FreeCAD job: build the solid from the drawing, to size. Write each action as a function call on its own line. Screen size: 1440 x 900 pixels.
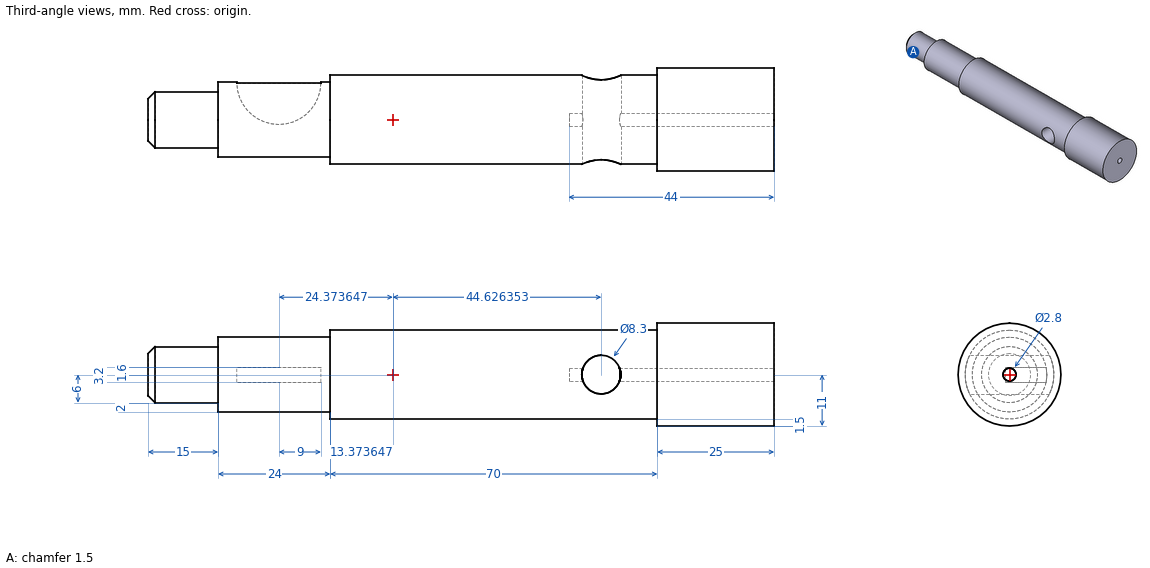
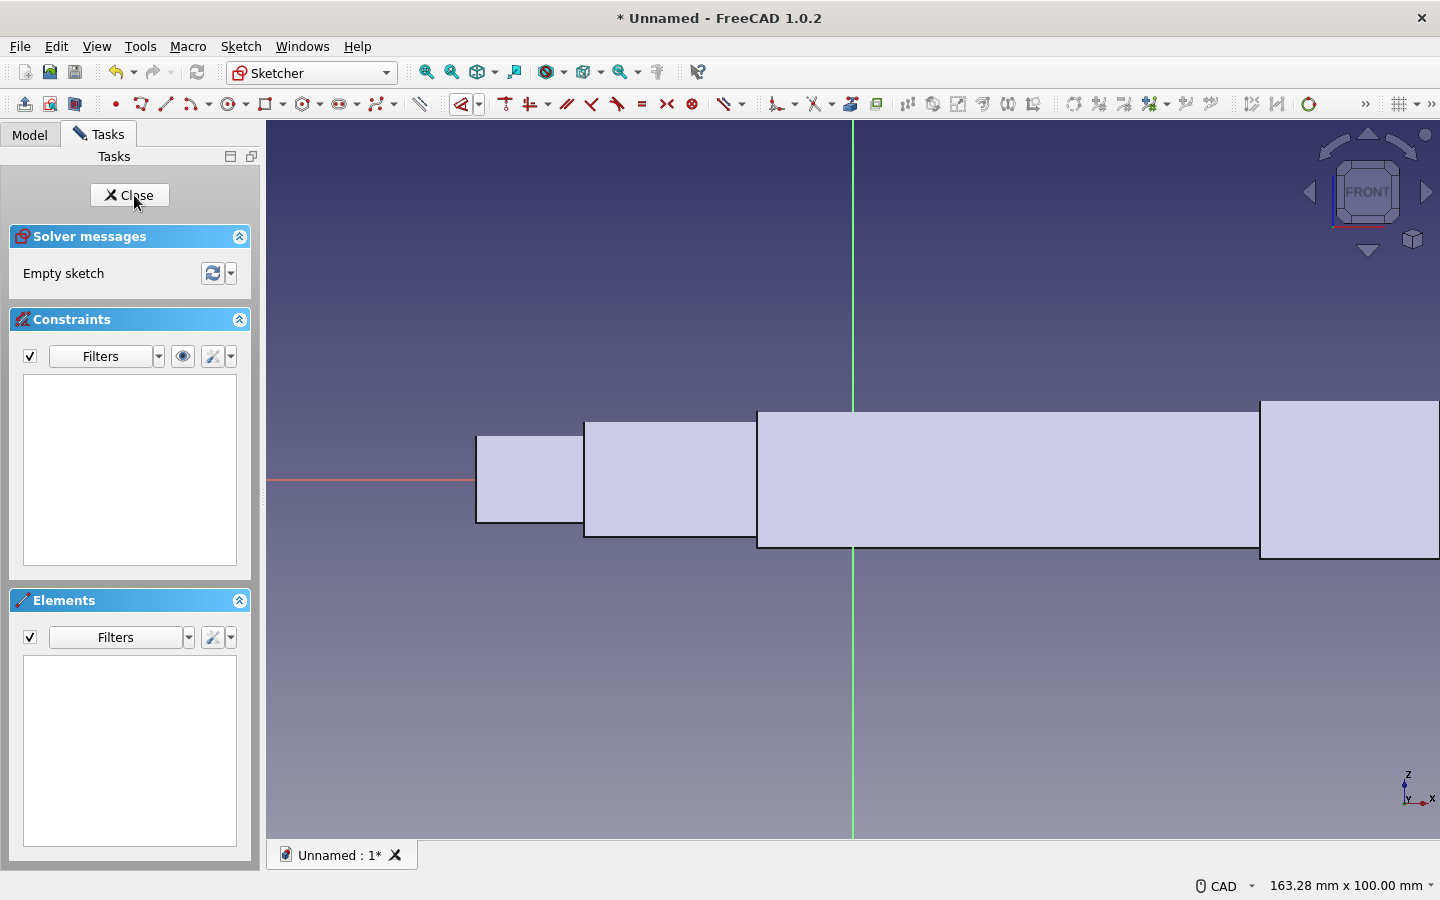
click(75, 104)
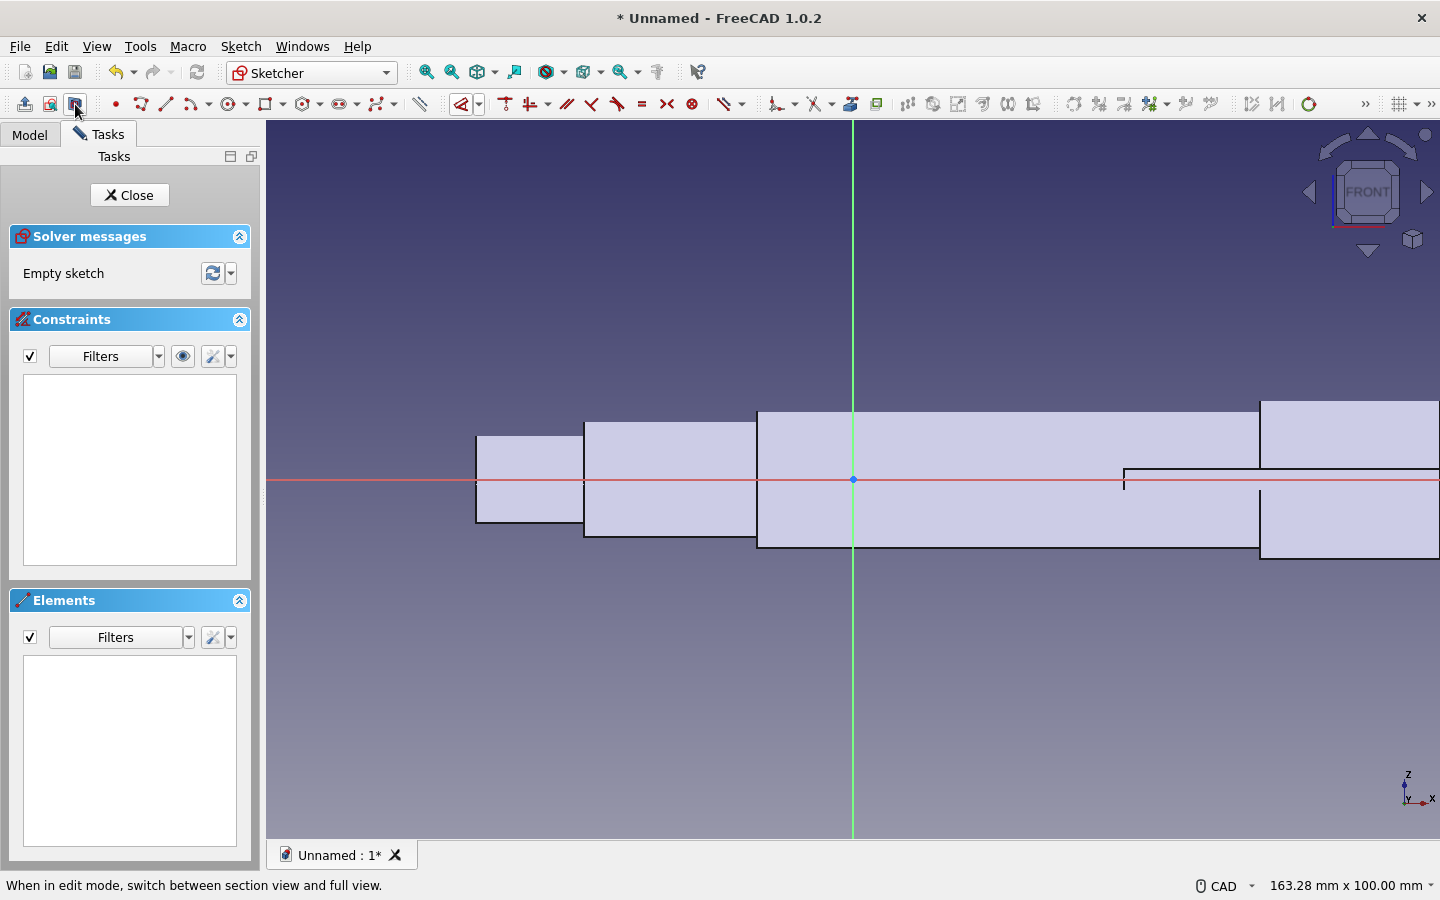
scroll(1235, 480, up, 10)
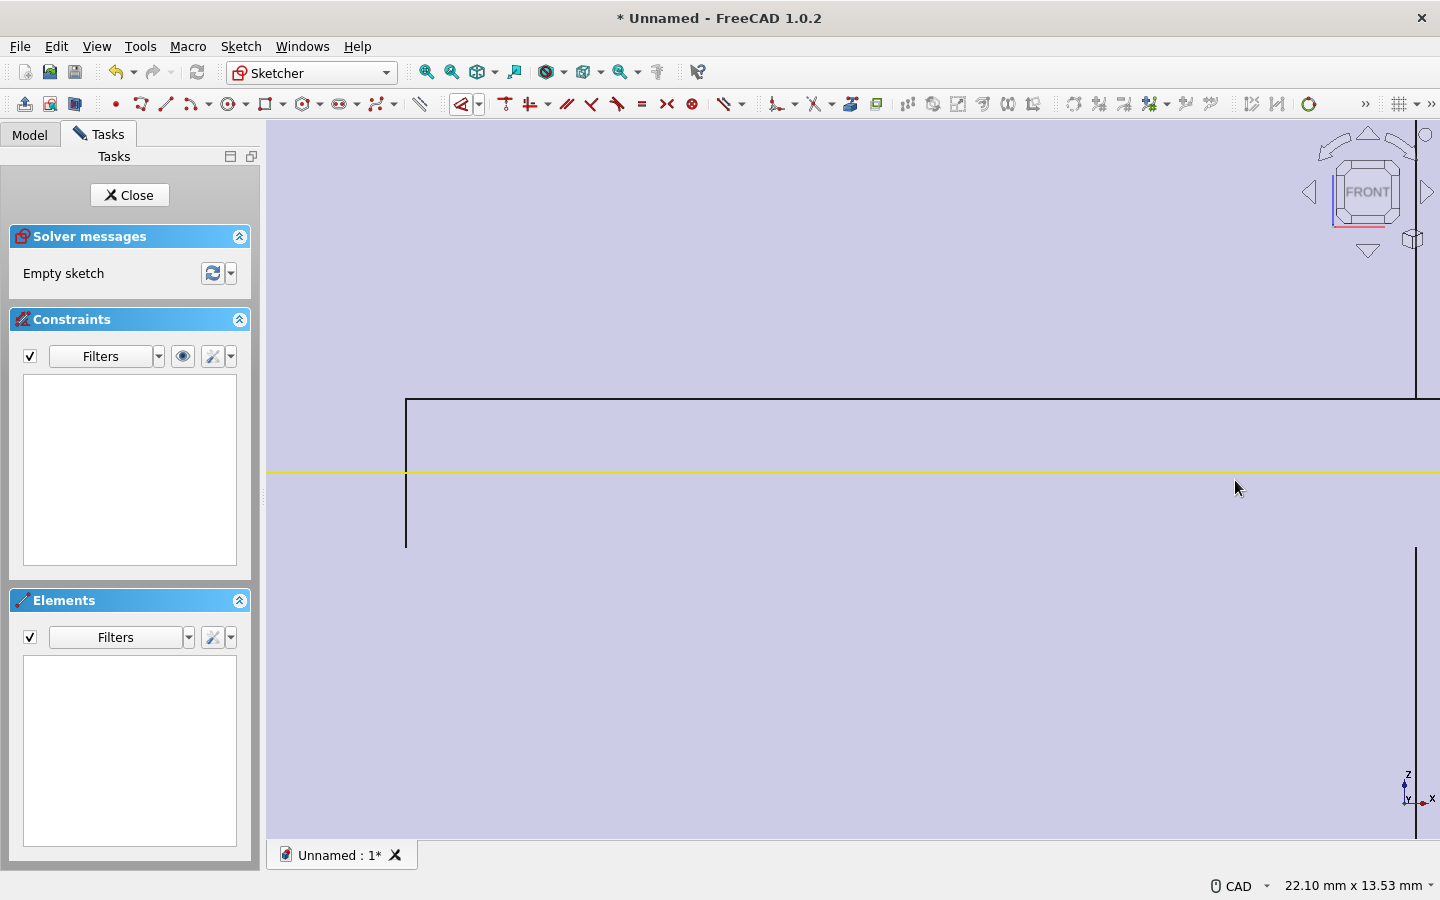
click(228, 104)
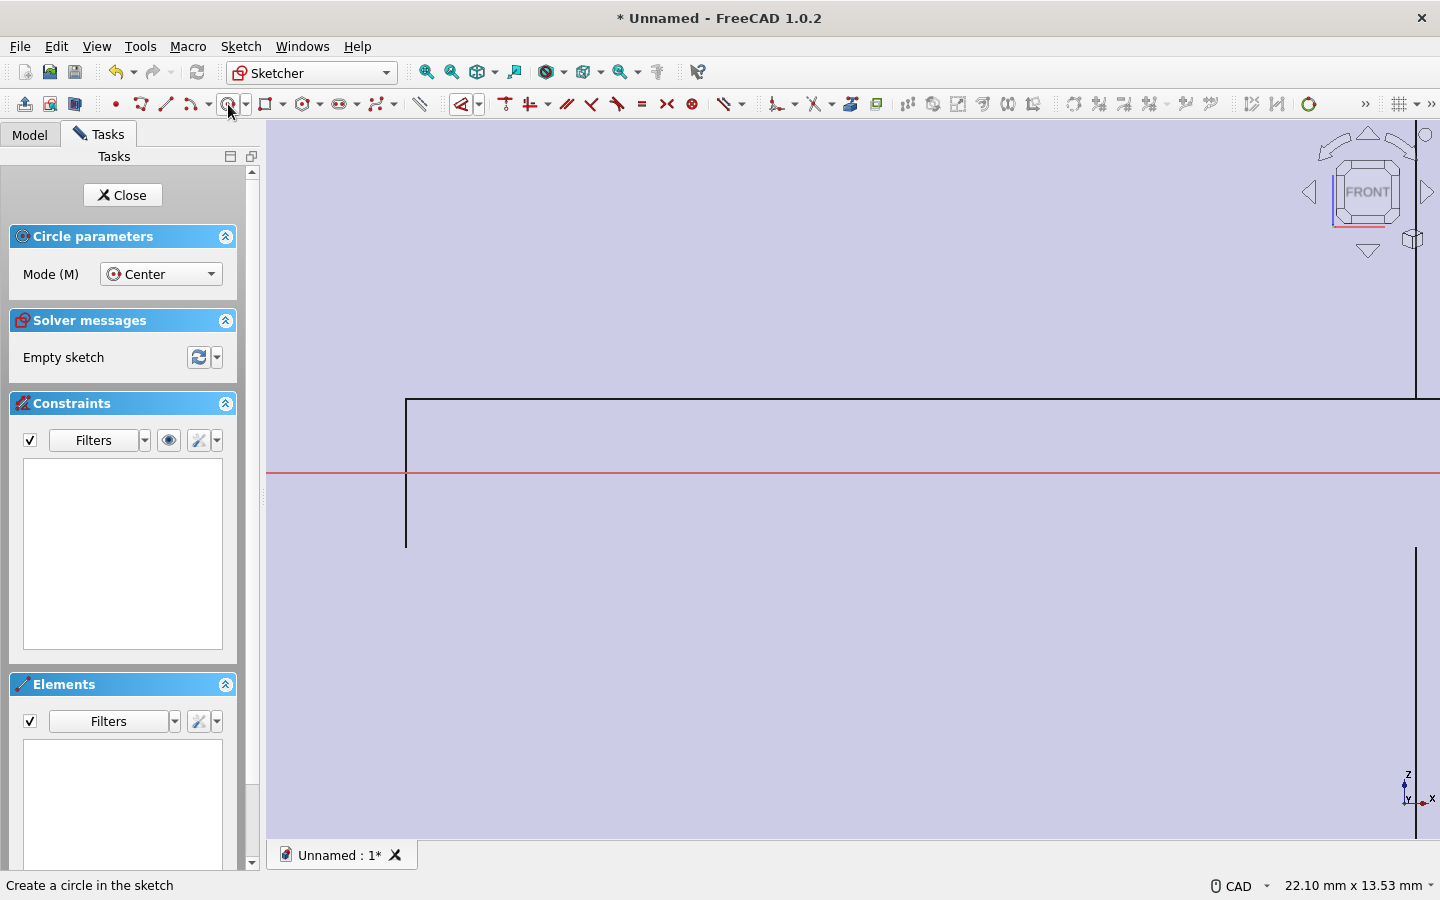
click(778, 473)
click(934, 317)
key(Escape)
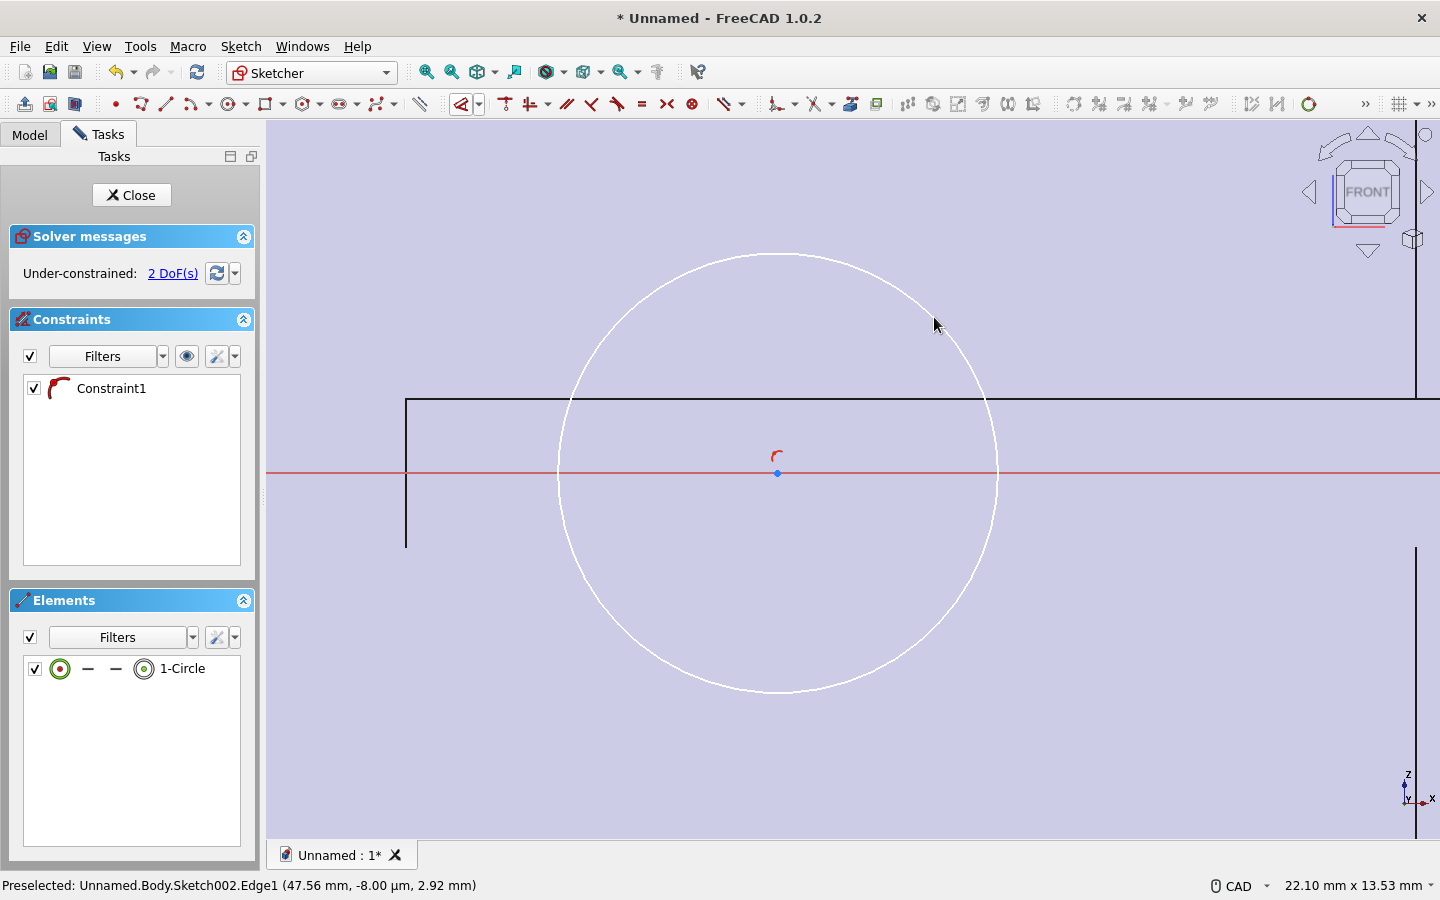
click(933, 317)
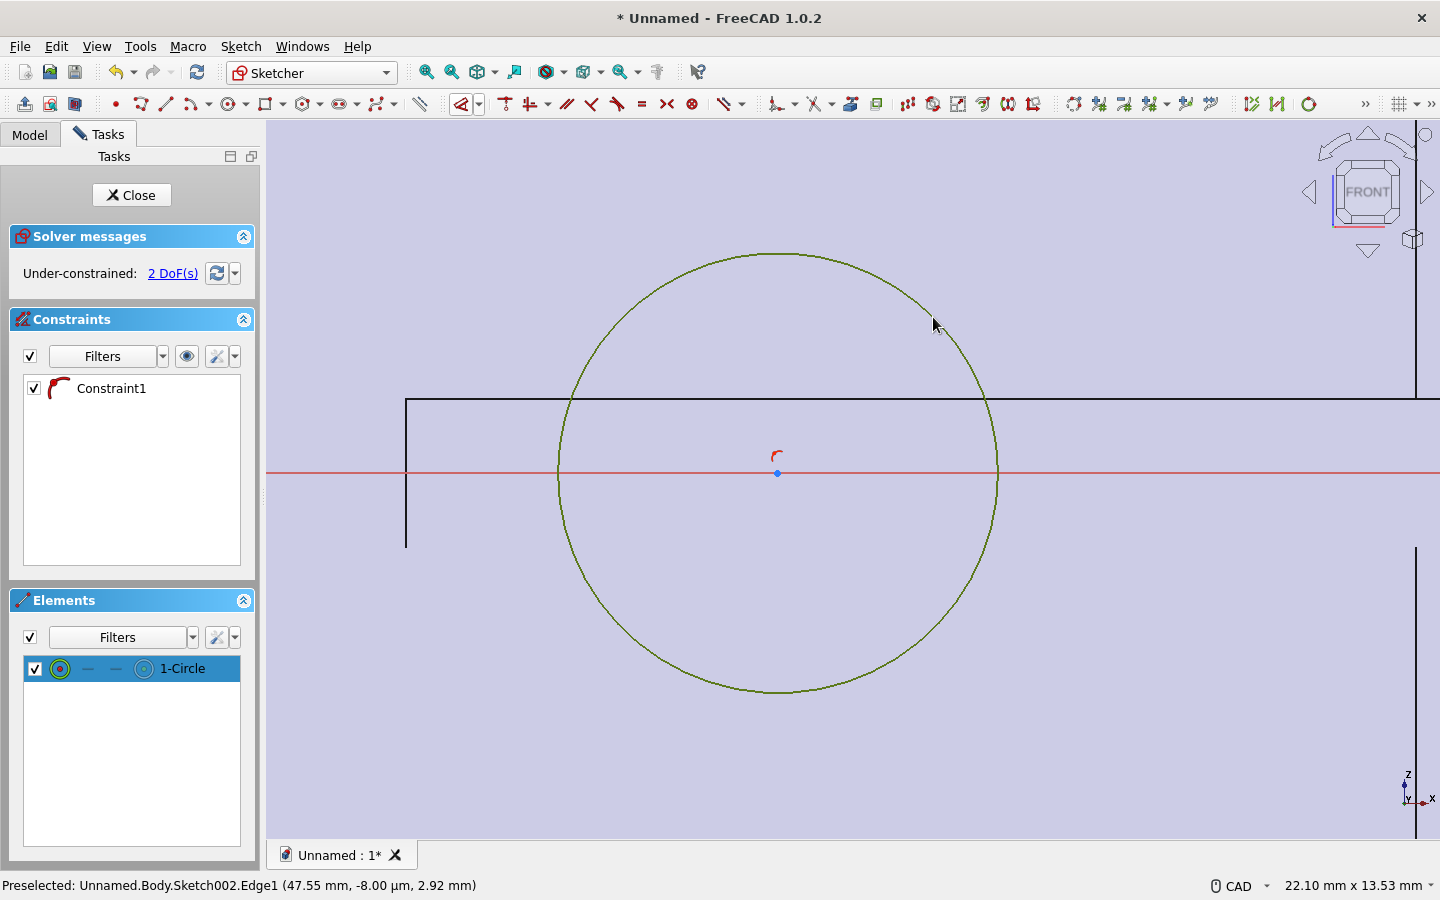
click(478, 104)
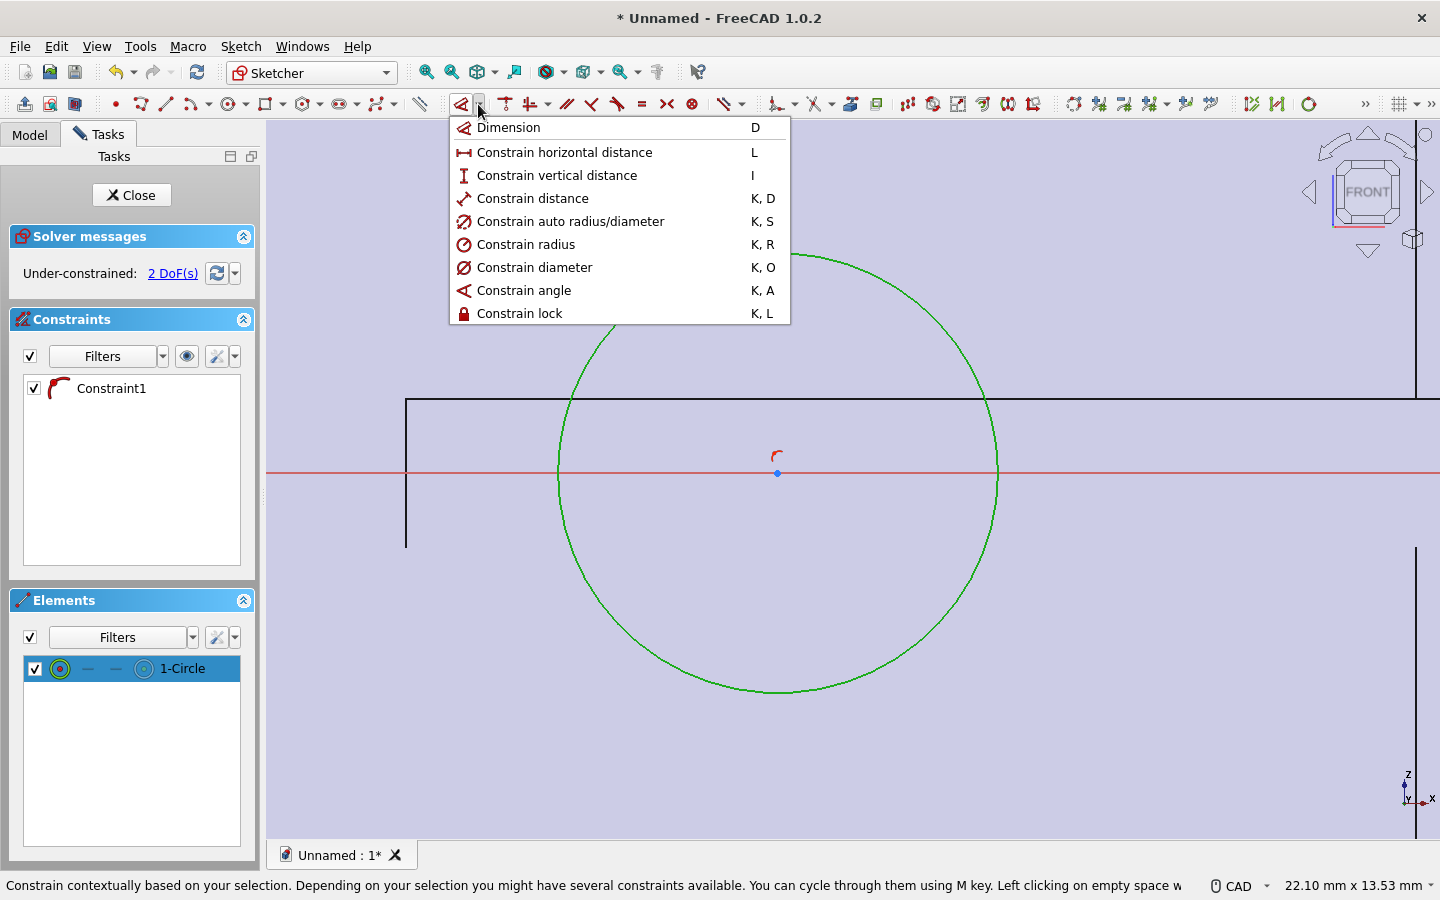
click(620, 268)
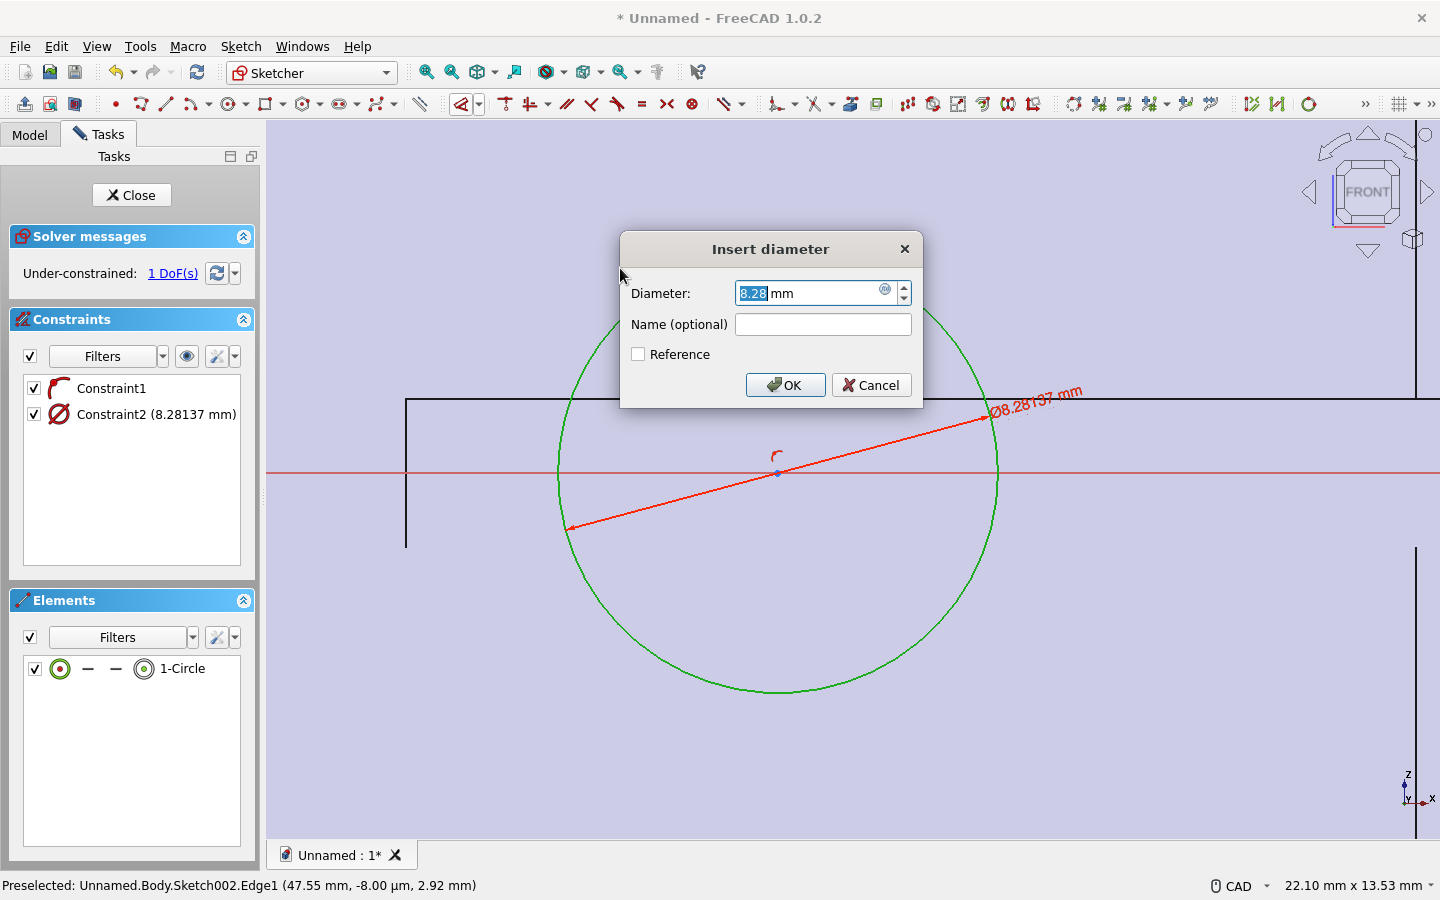
text(8.3)
key(Return)